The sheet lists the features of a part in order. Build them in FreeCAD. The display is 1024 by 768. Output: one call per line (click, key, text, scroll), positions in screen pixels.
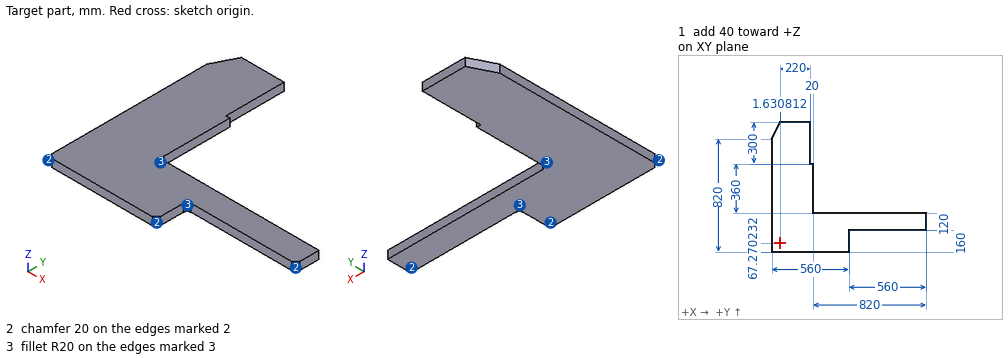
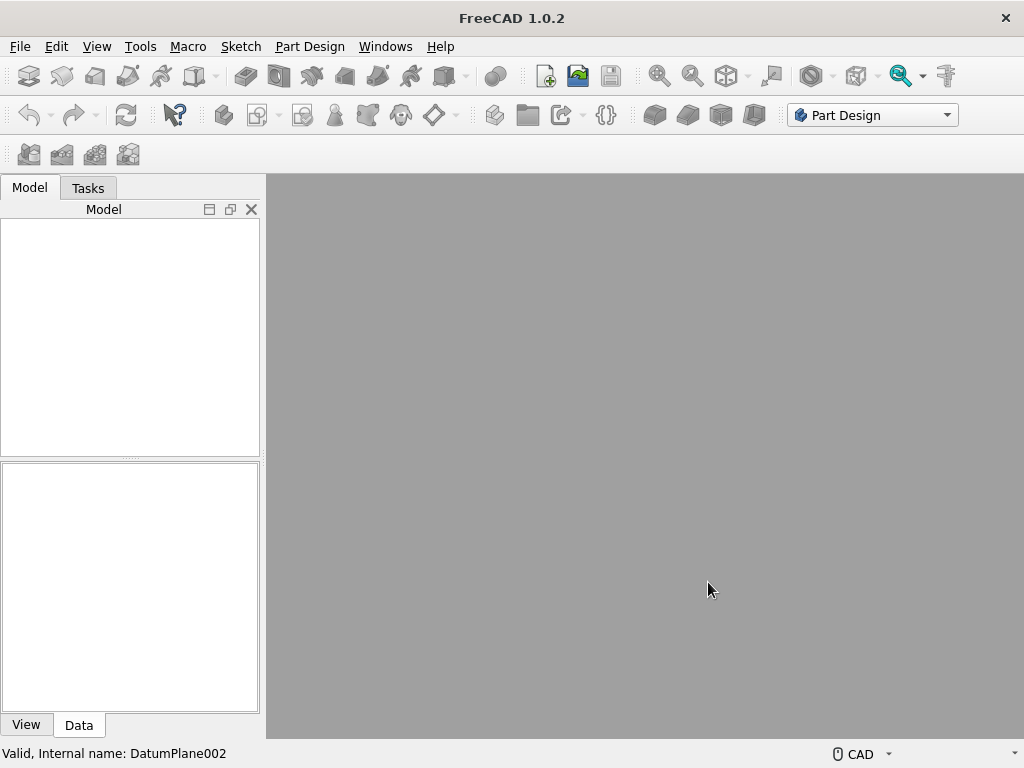
key(ctrl+n)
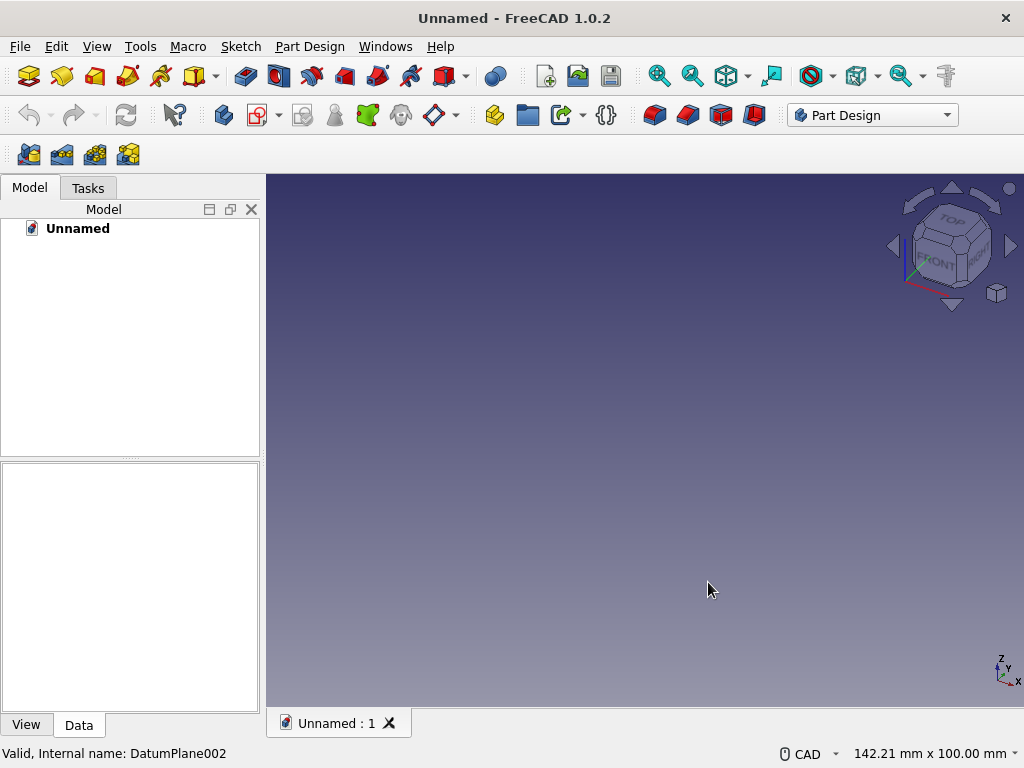
click(256, 116)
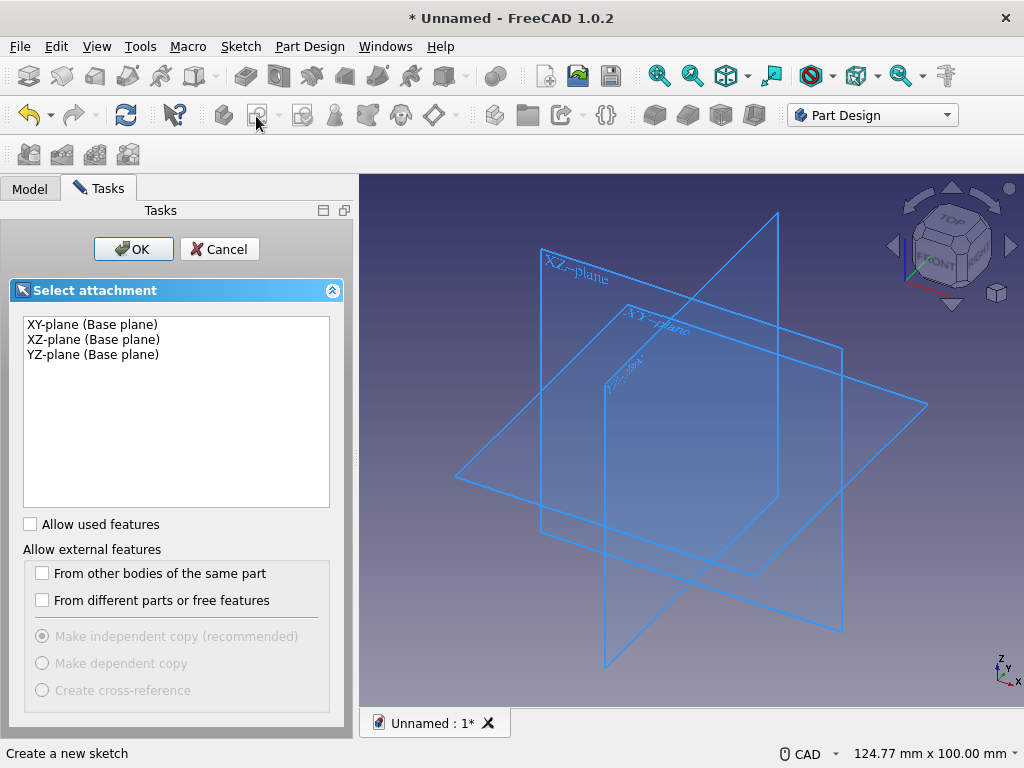
click(84, 324)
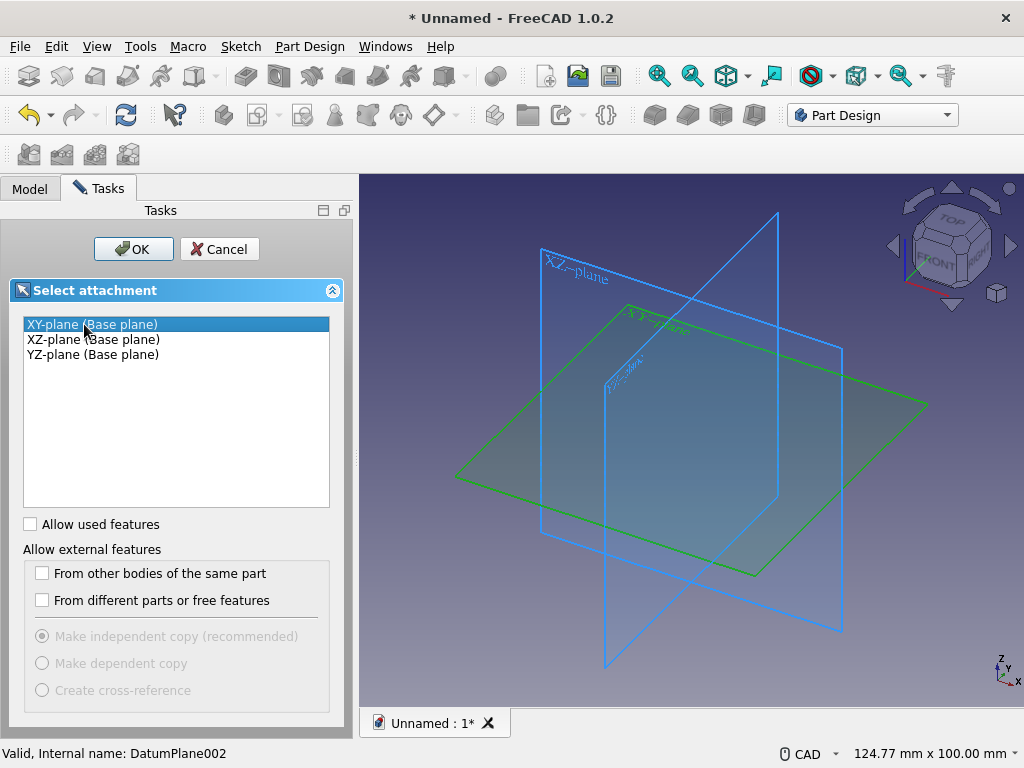
click(134, 249)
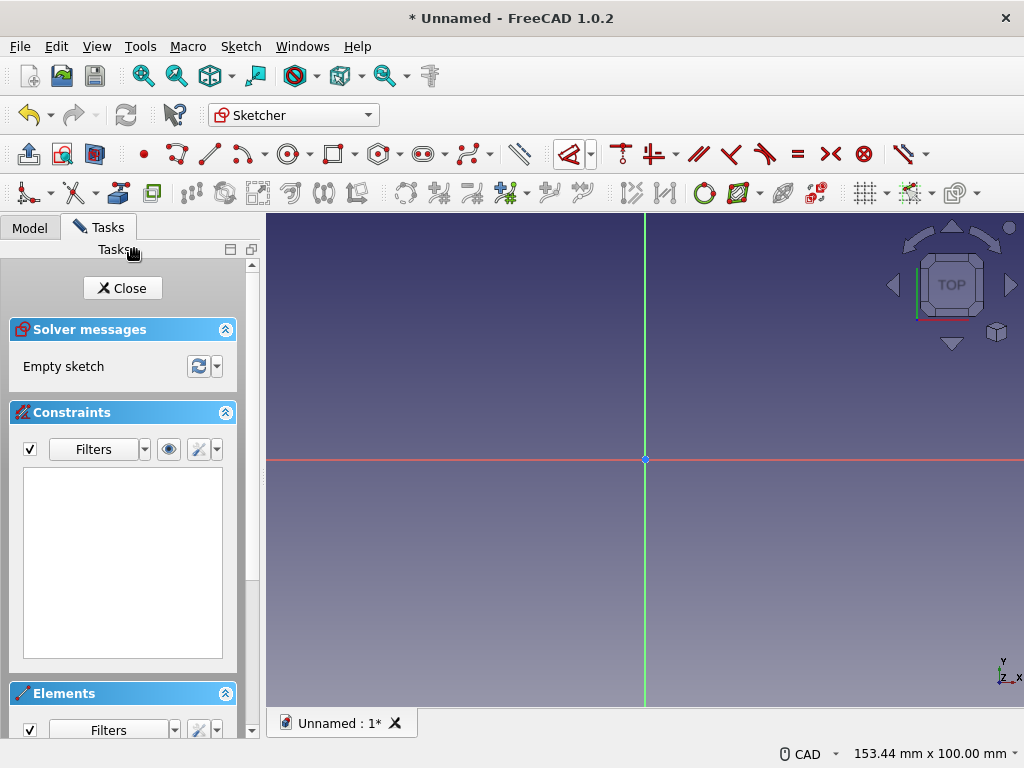
scroll(413, 589, down, 14)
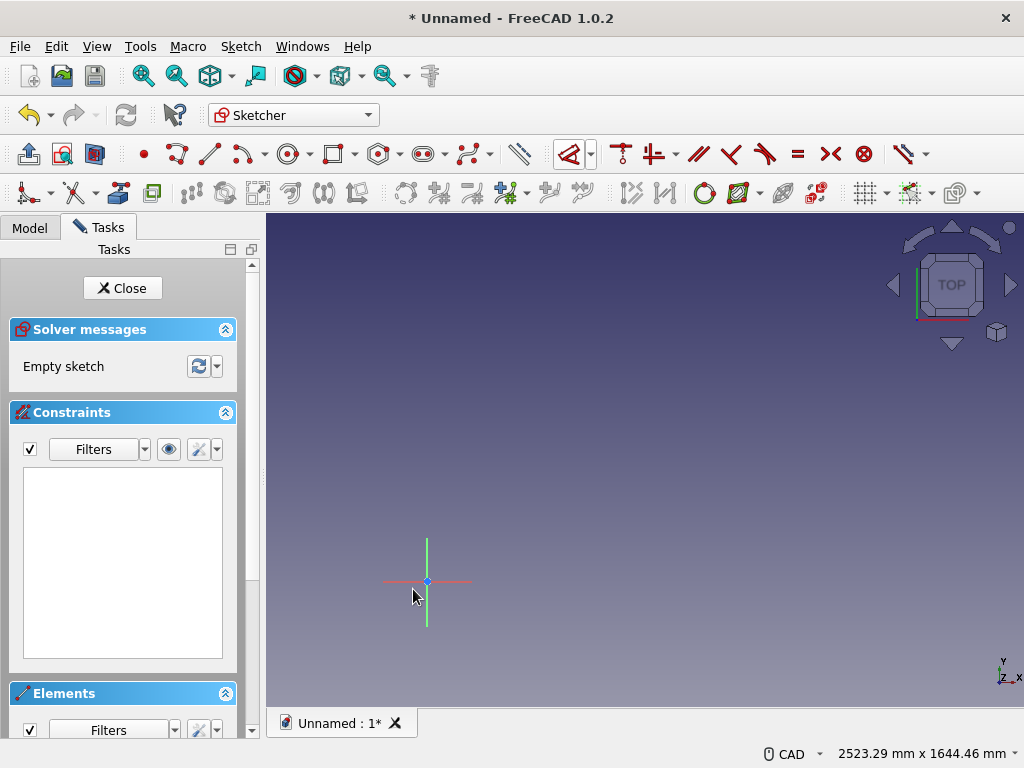
key(g)
key(m)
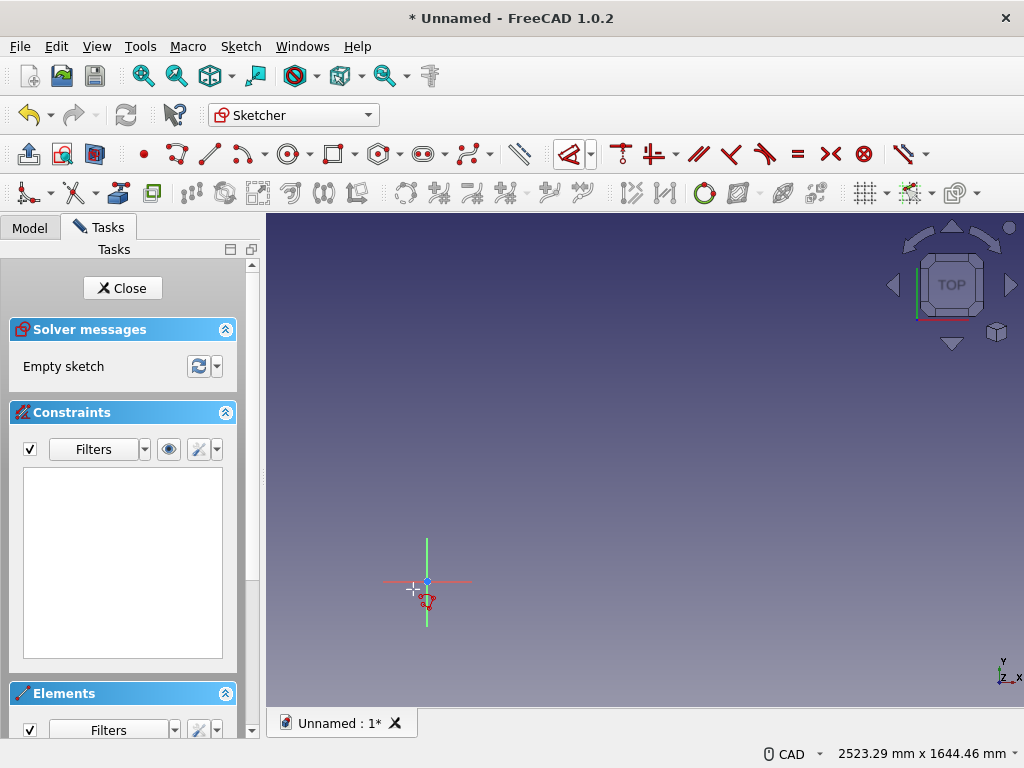
click(409, 602)
click(577, 602)
click(577, 554)
click(745, 554)
click(745, 518)
click(499, 518)
click(499, 410)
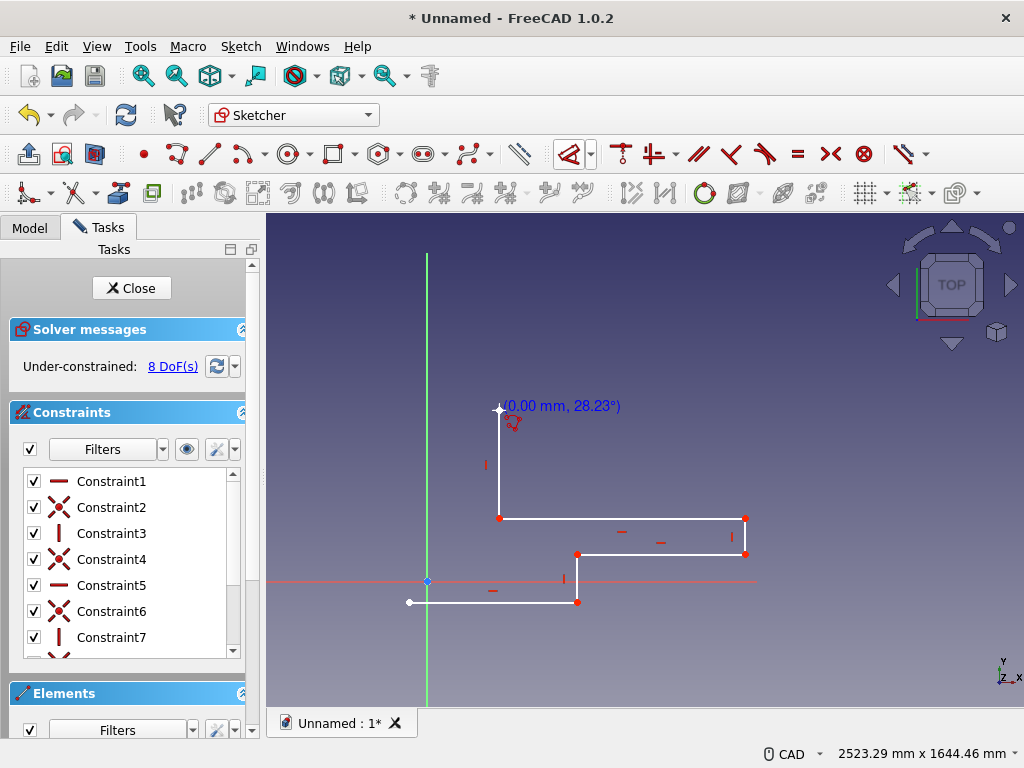
scroll(493, 410, up, 5)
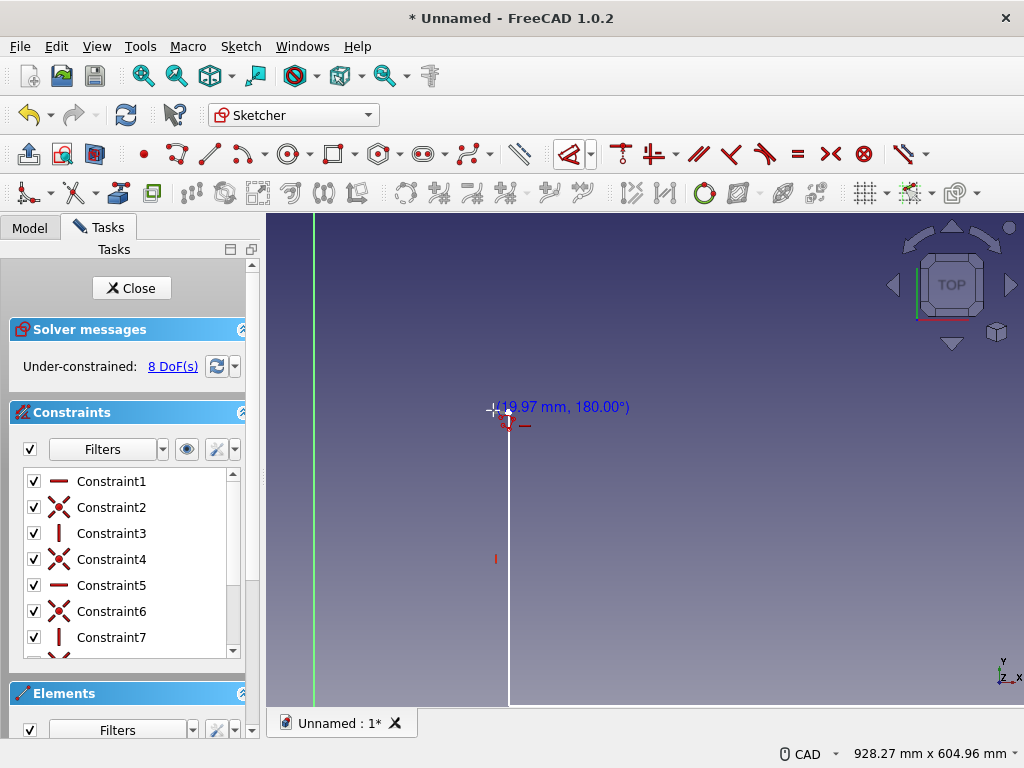
click(492, 409)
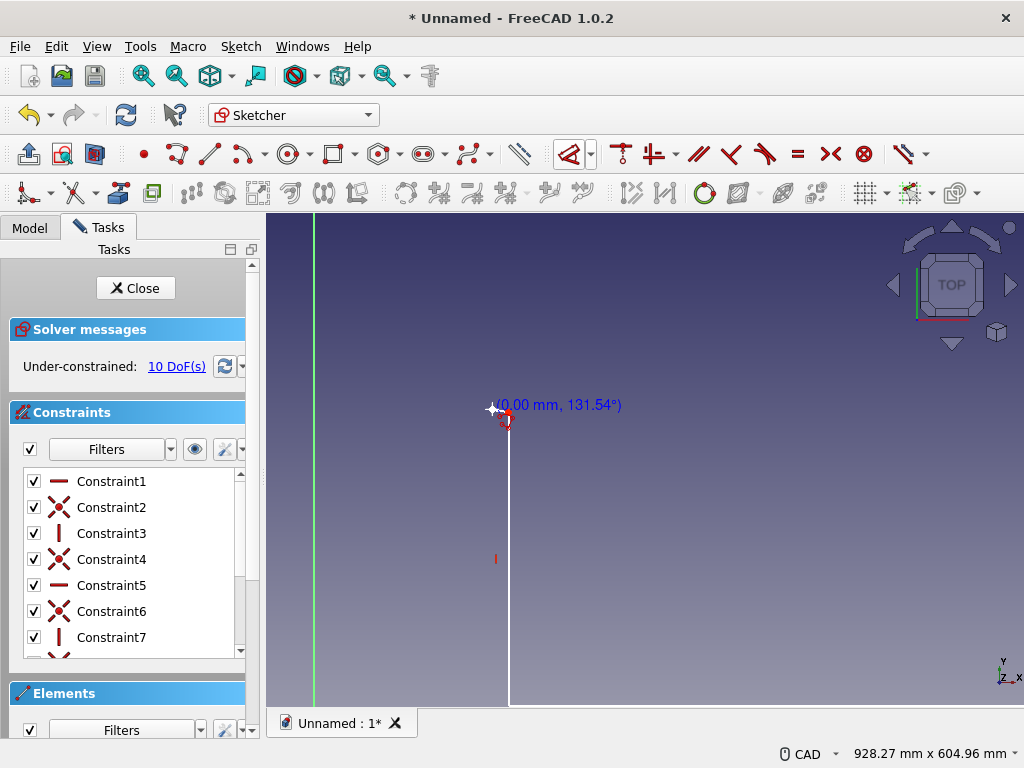
scroll(493, 409, down, 5)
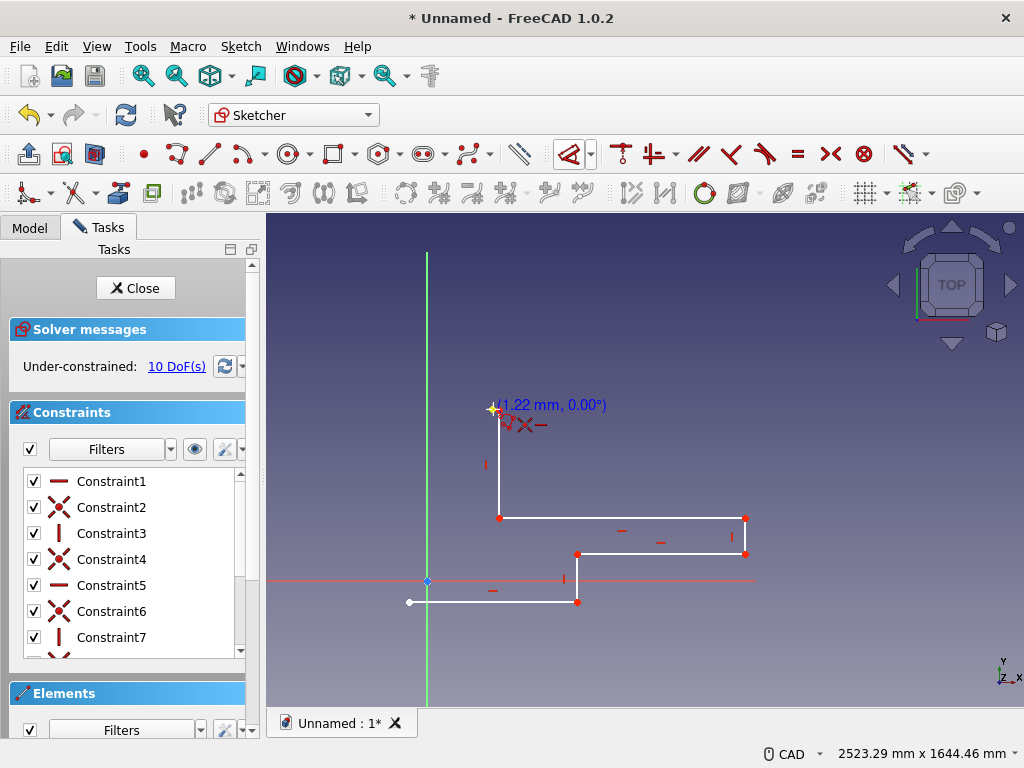
click(493, 319)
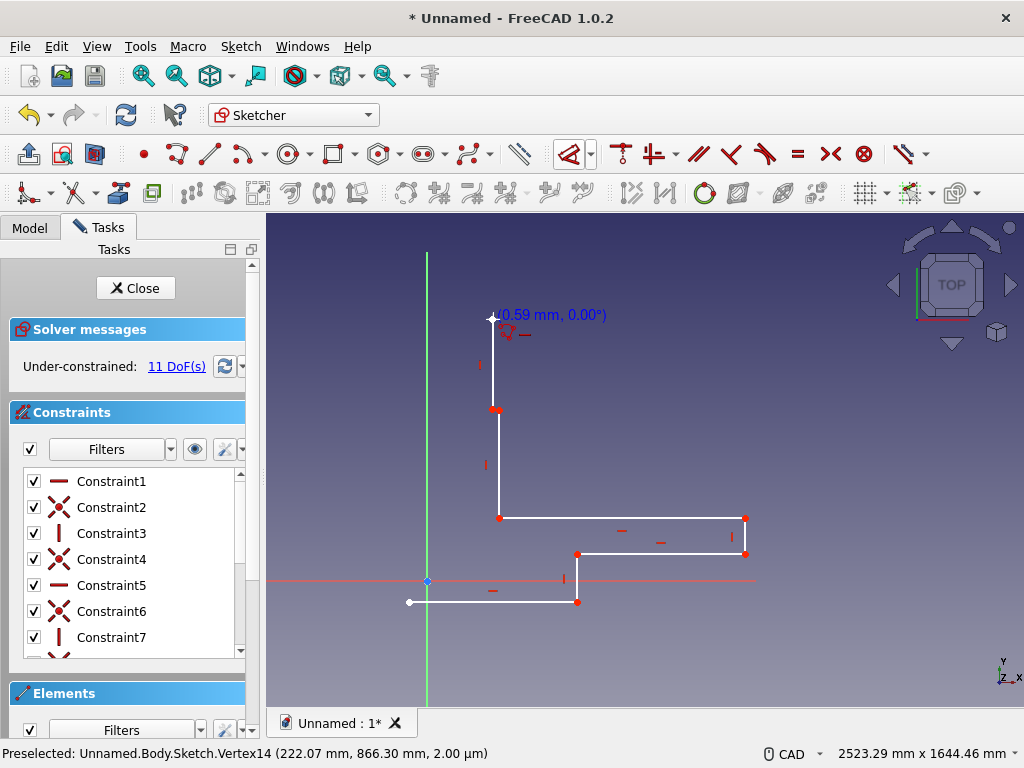
scroll(427, 319, up, 18)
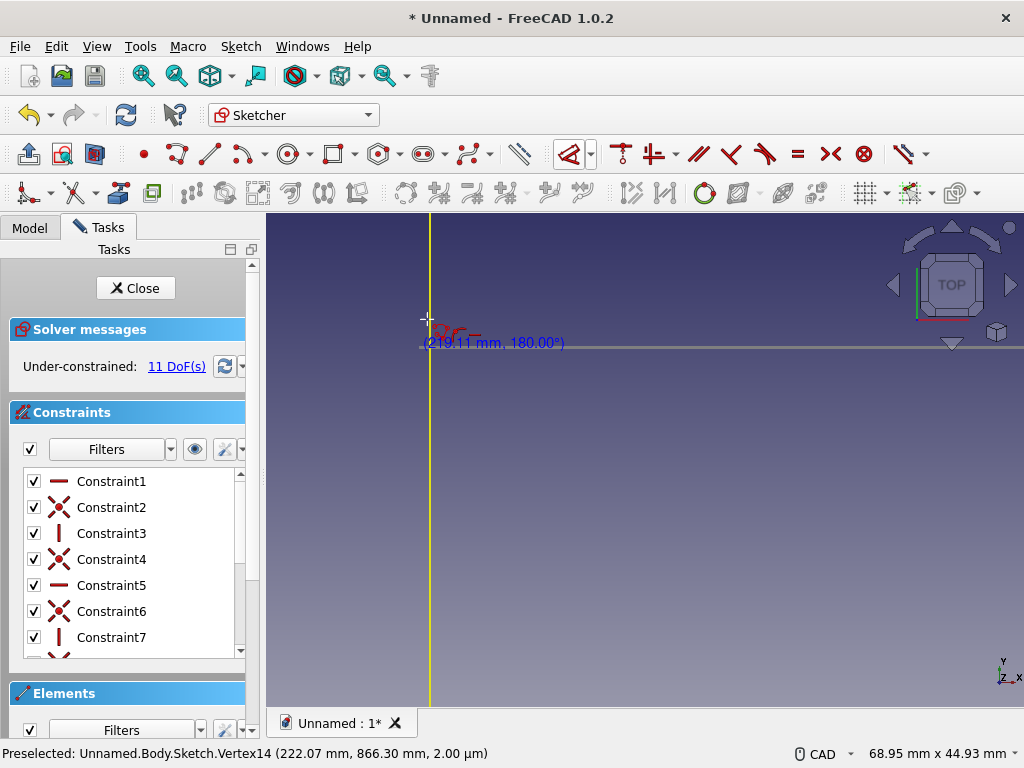
click(412, 311)